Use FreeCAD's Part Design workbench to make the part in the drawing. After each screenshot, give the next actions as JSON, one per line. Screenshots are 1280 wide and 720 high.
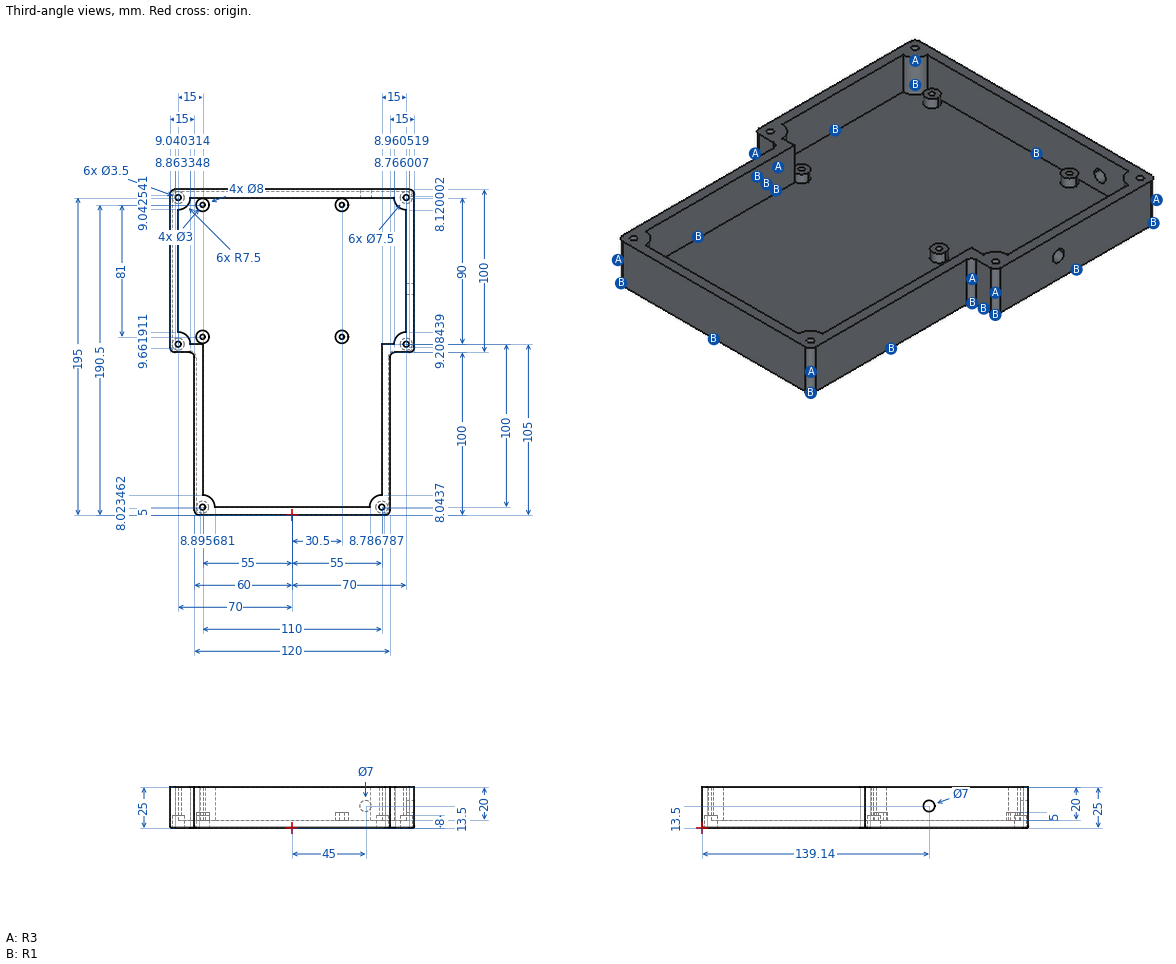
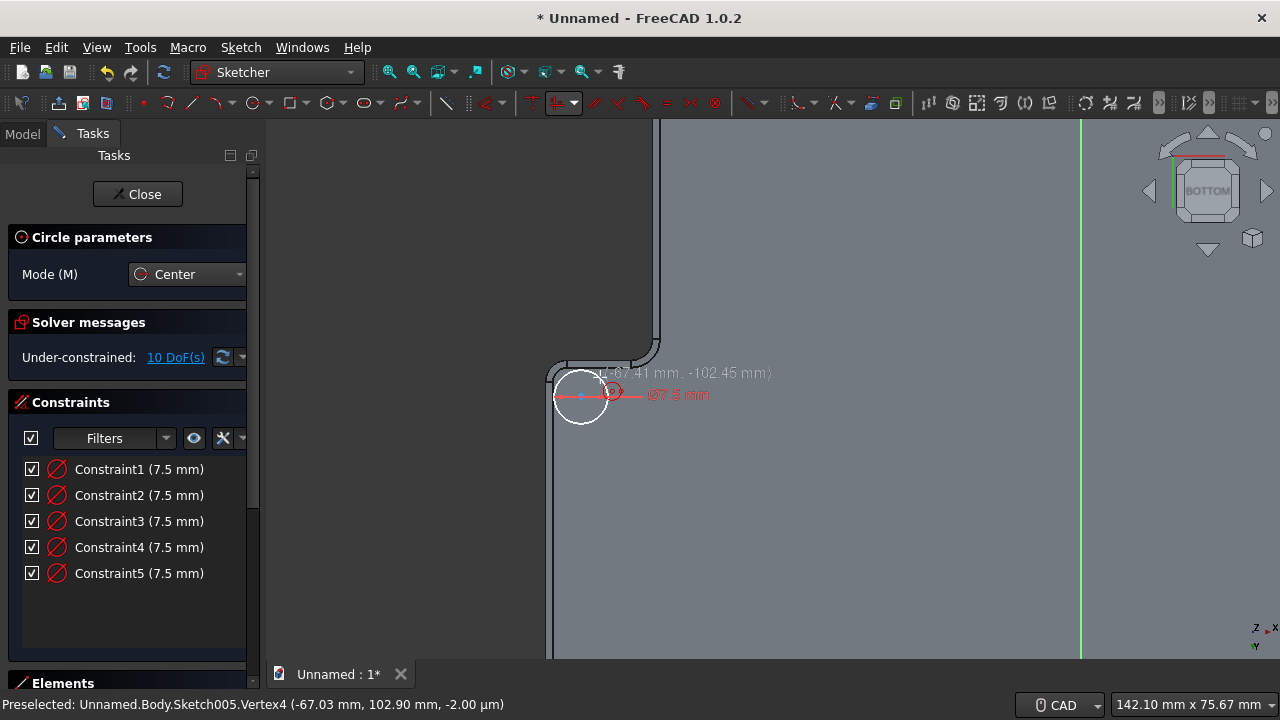
{"action": "scroll", "coordinate": [581, 400], "scroll_direction": "down", "scroll_amount": 7}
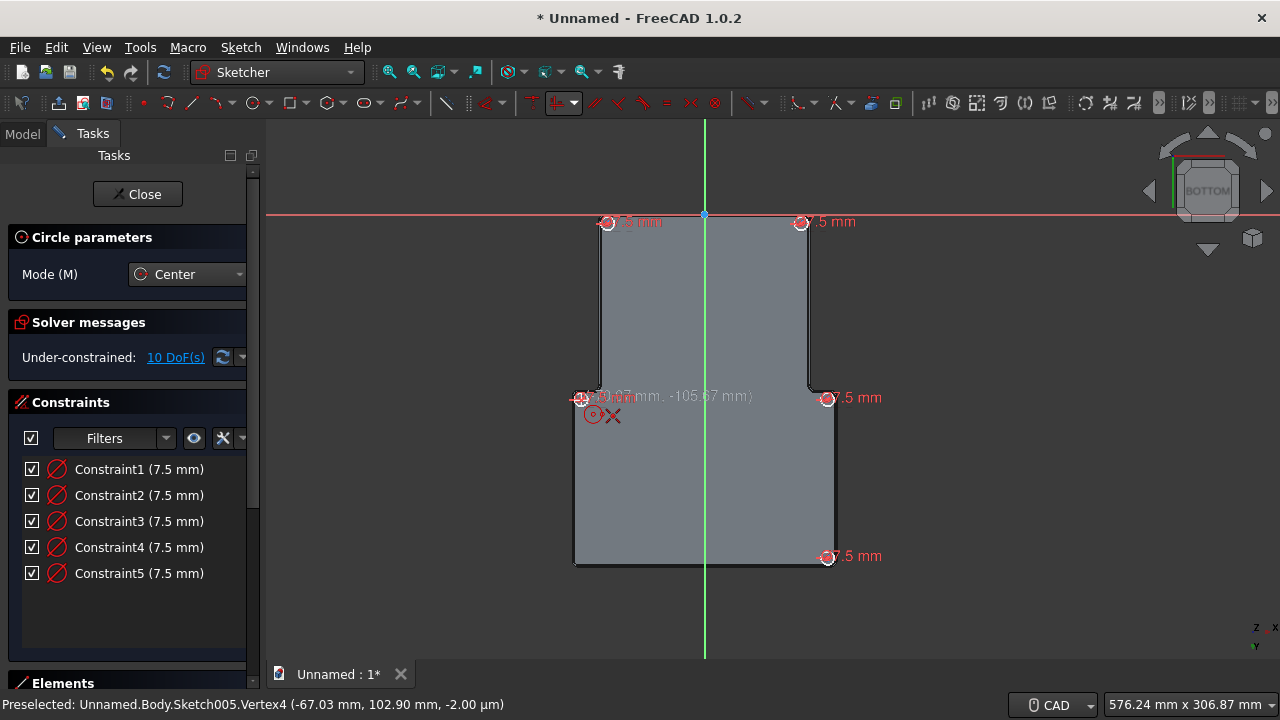
{"action": "scroll", "coordinate": [581, 558], "scroll_direction": "up", "scroll_amount": 7}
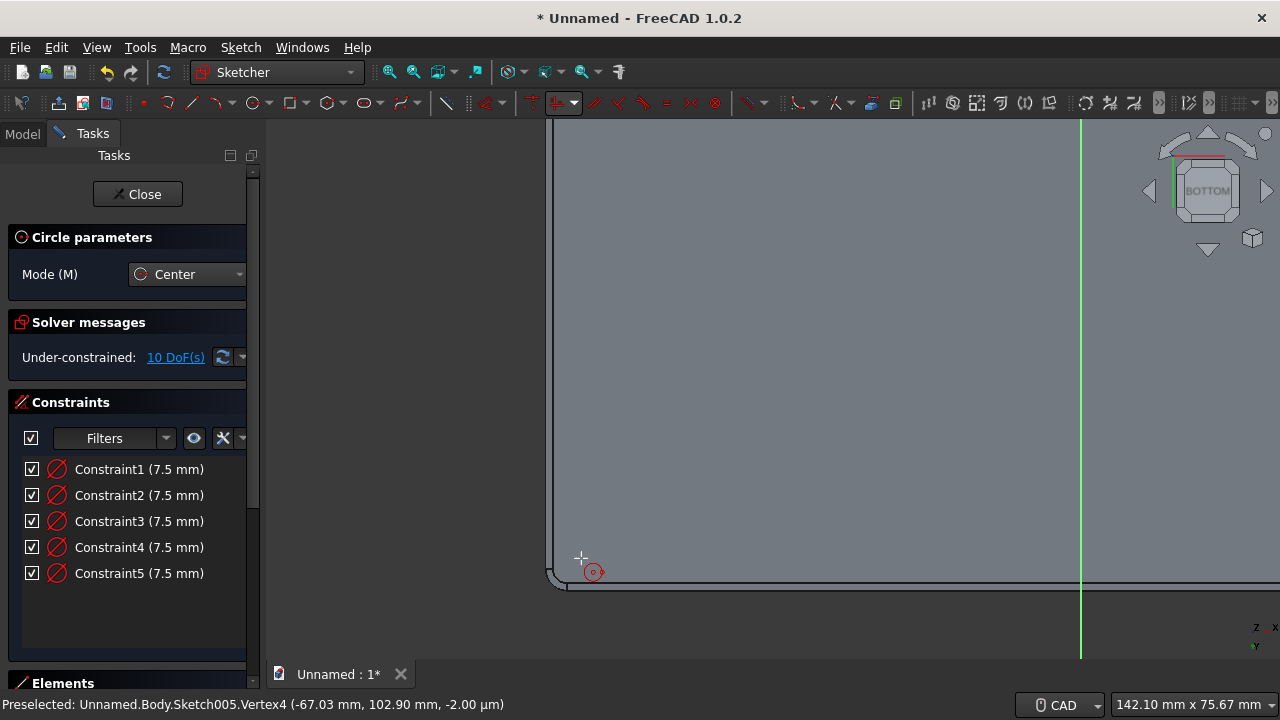
{"action": "left_click", "coordinate": [581, 555]}
{"action": "mouse_move", "coordinate": [600, 536]}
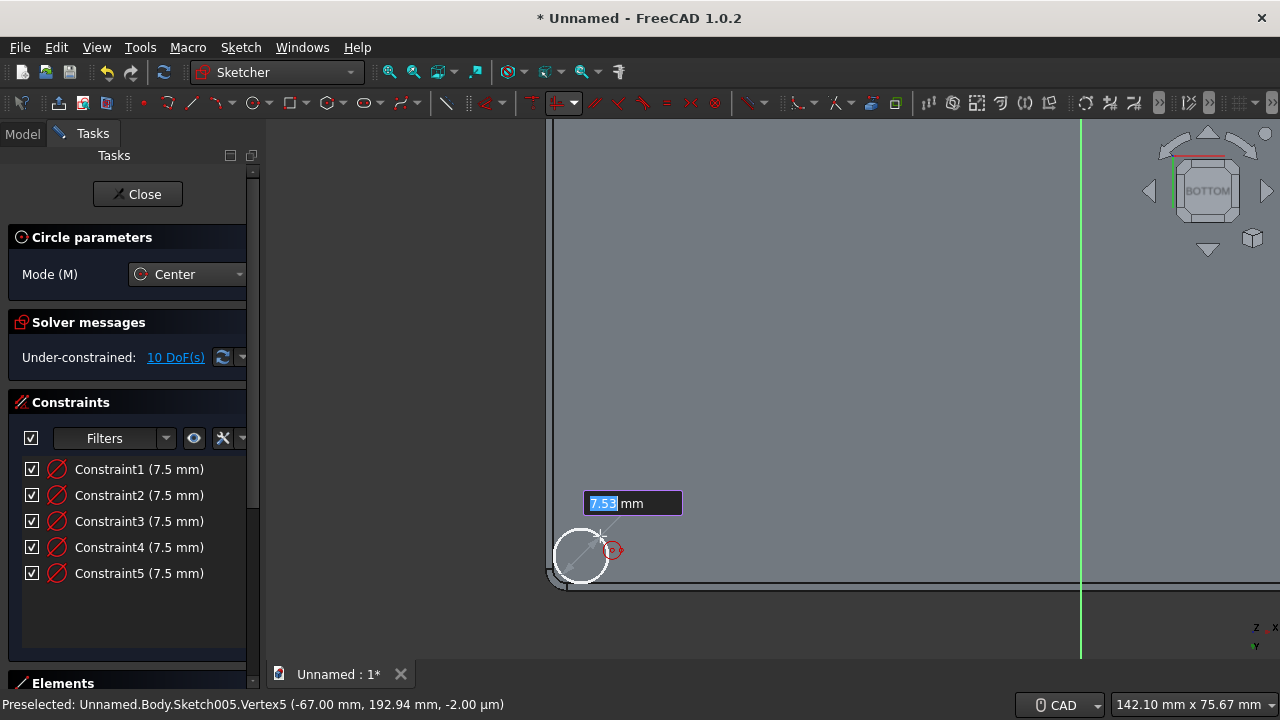
{"action": "type", "text": "7.5"}
{"action": "key", "text": "Return"}
{"action": "key", "text": "Escape"}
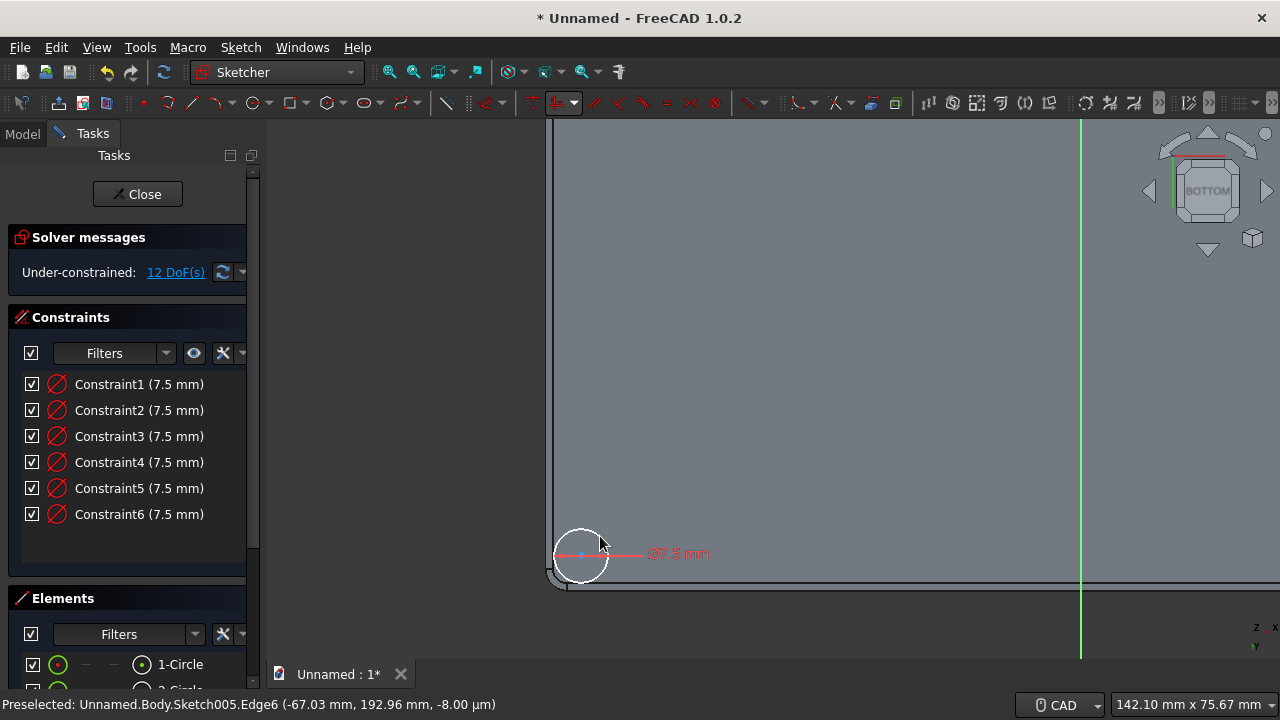
{"action": "scroll", "coordinate": [581, 558], "scroll_direction": "down", "scroll_amount": 7}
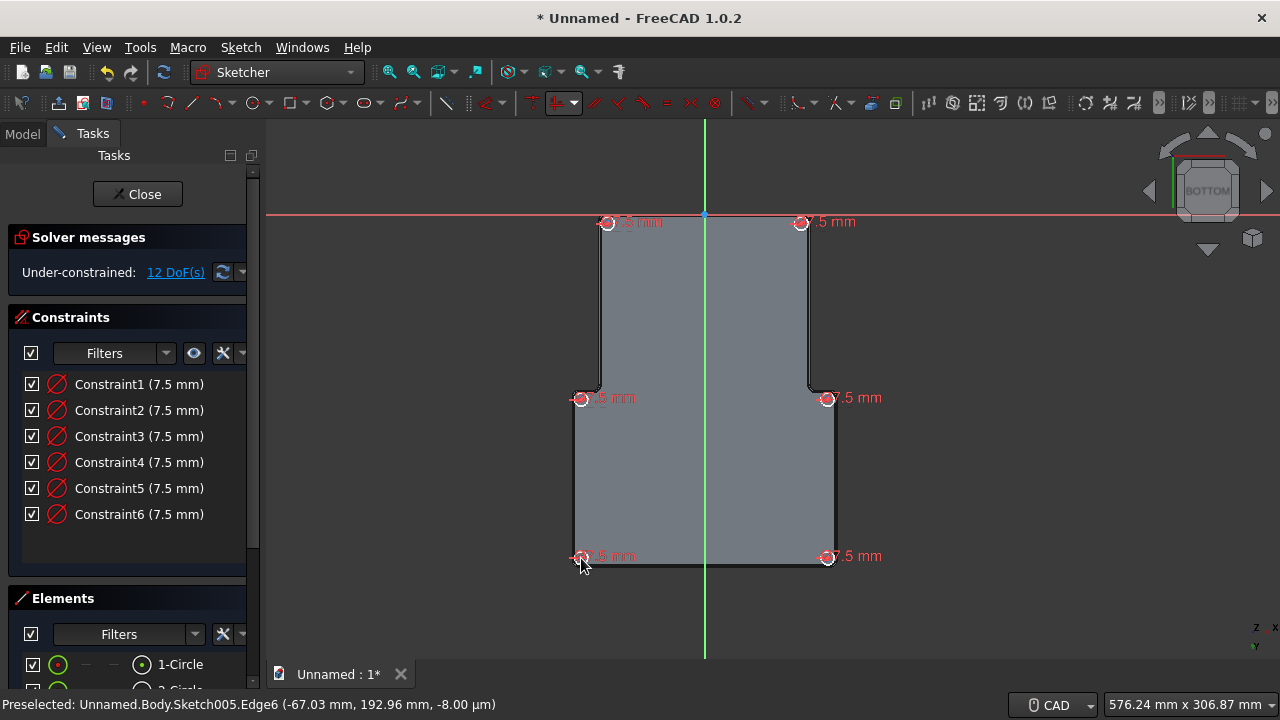
{"action": "left_click", "coordinate": [828, 558]}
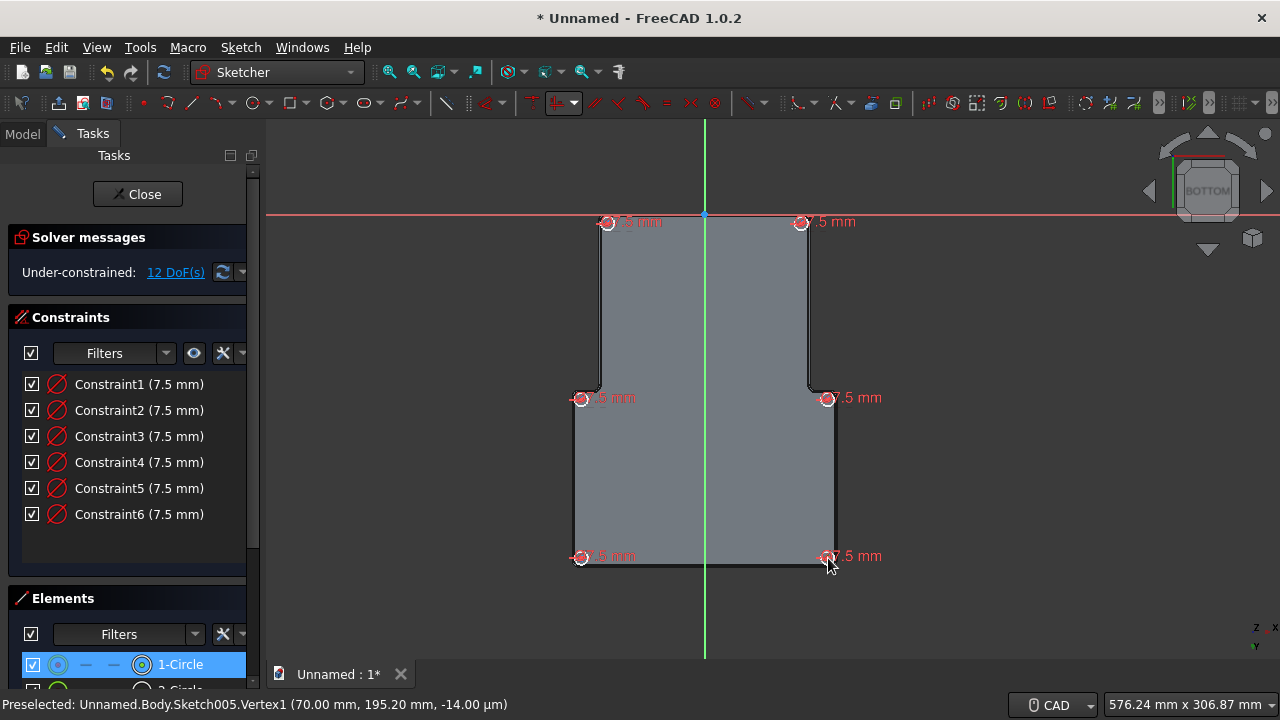
{"action": "left_click", "coordinate": [828, 400]}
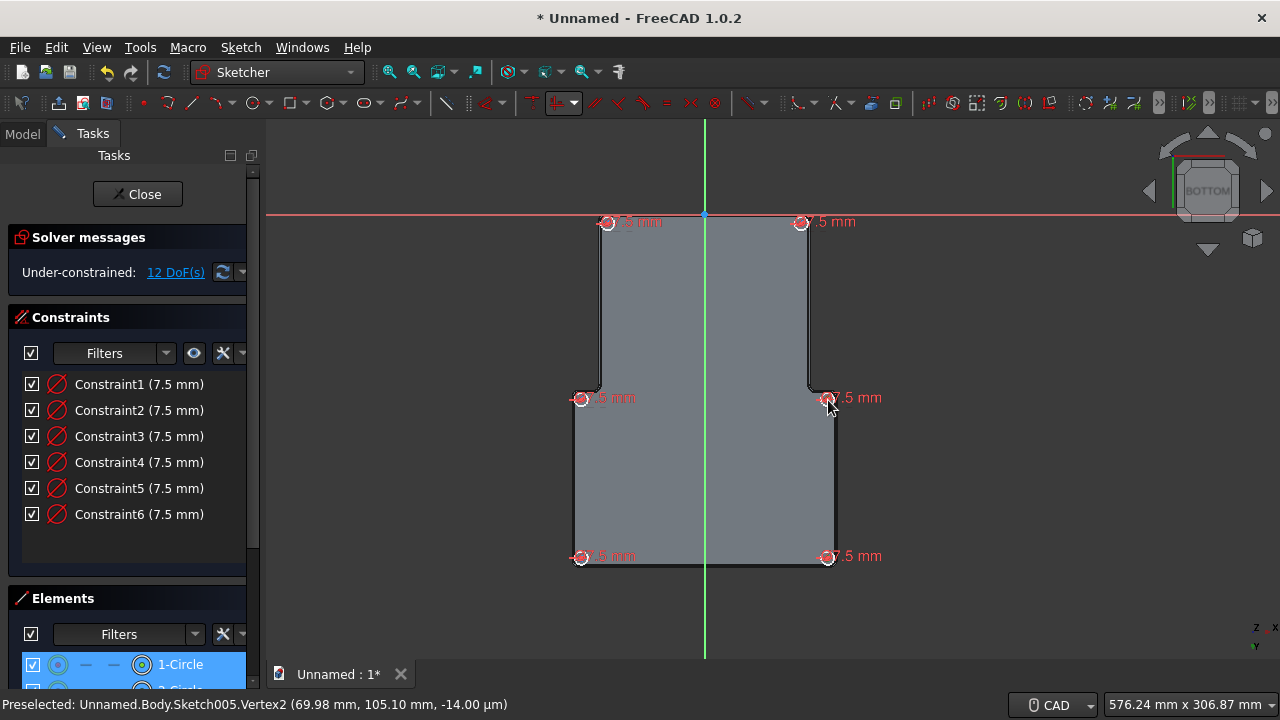
{"action": "key", "text": "v"}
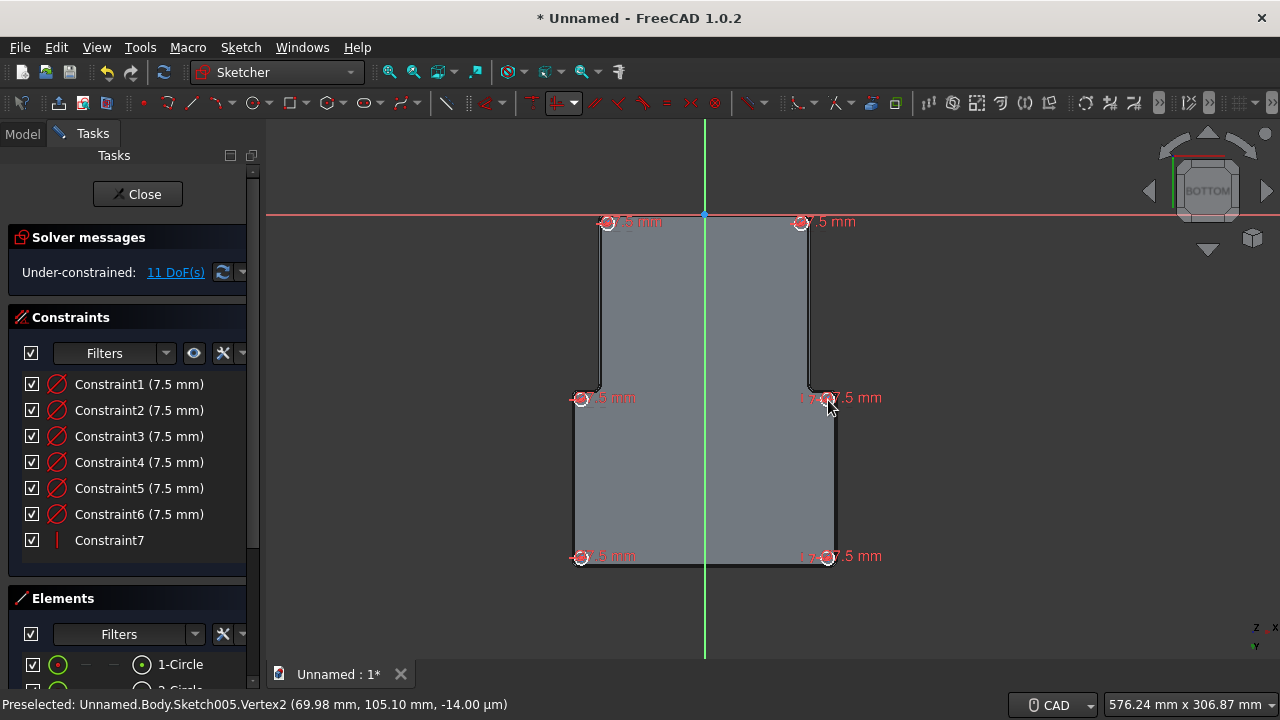
{"action": "left_click", "coordinate": [801, 224]}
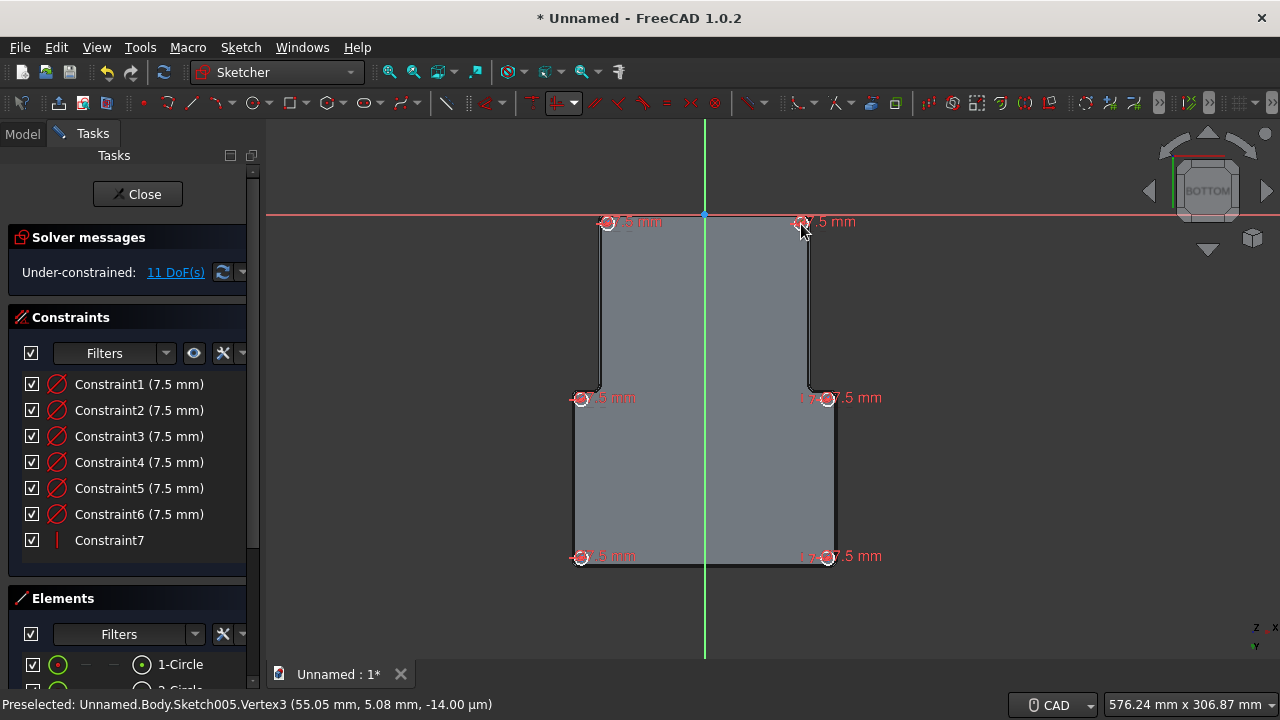
{"action": "left_click", "coordinate": [608, 224]}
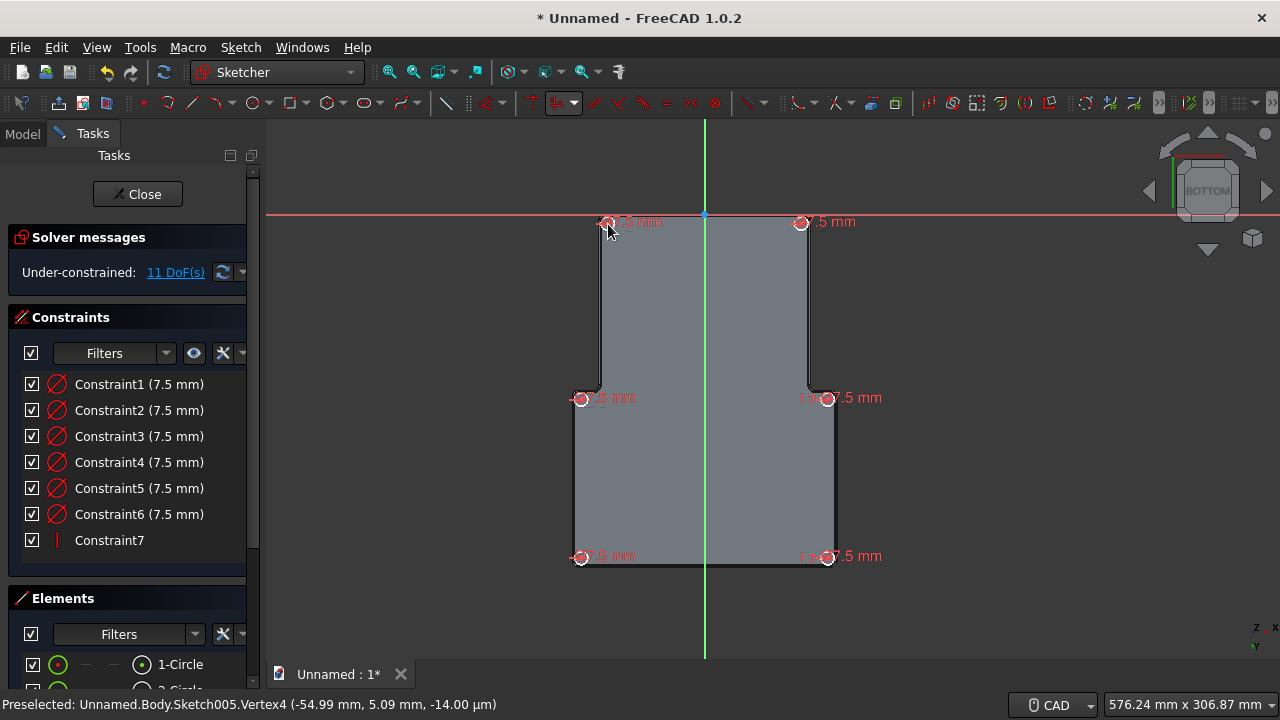
{"action": "key", "text": "h"}